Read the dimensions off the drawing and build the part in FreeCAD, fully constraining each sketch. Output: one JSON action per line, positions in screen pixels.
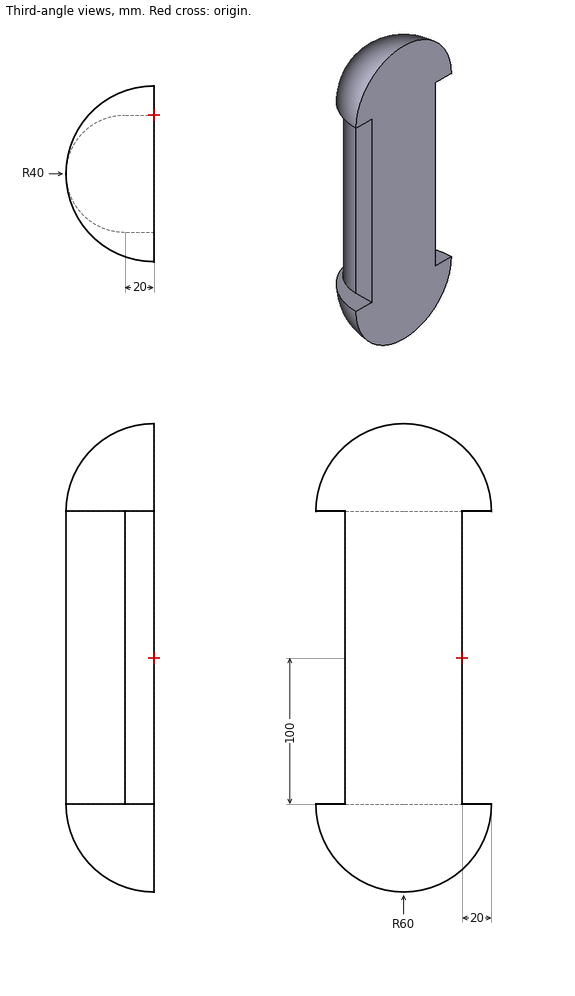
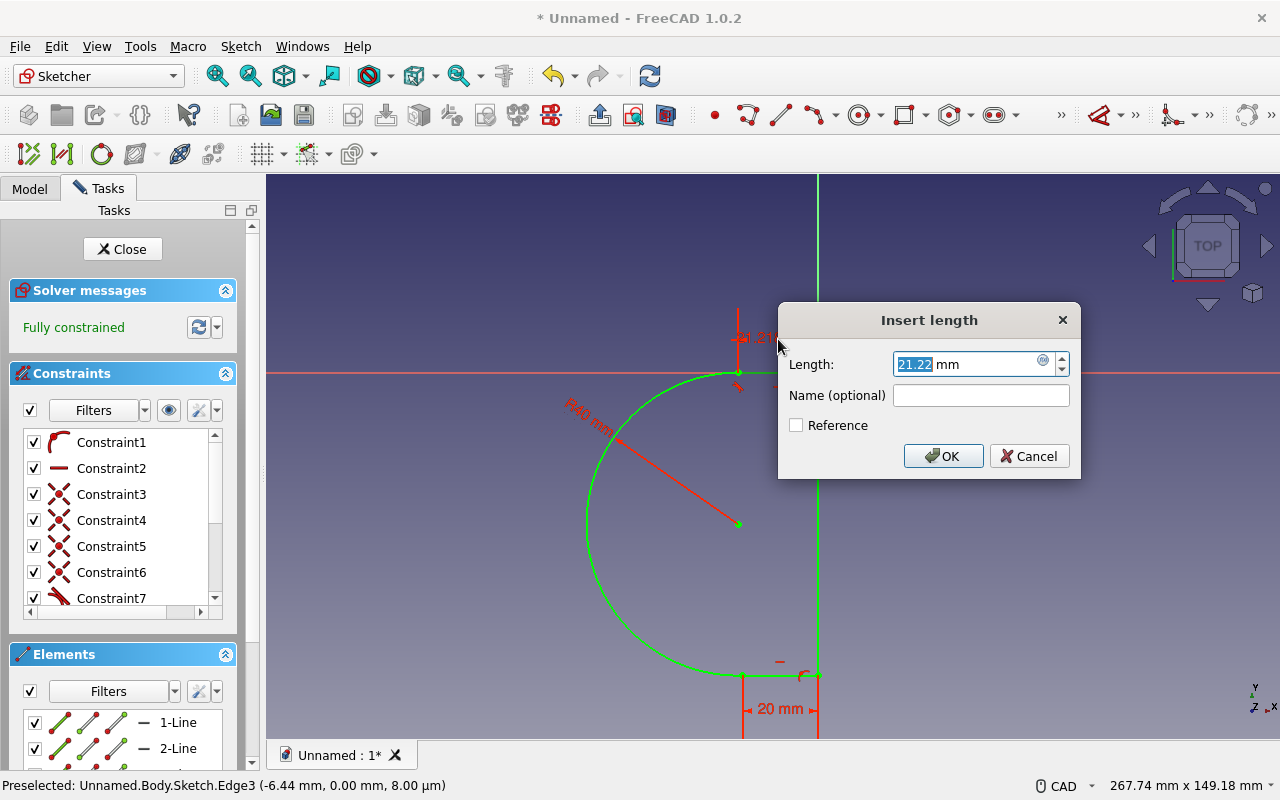
{"action": "type", "text": "20"}
{"action": "key", "text": "Return"}
{"action": "key", "text": "Escape"}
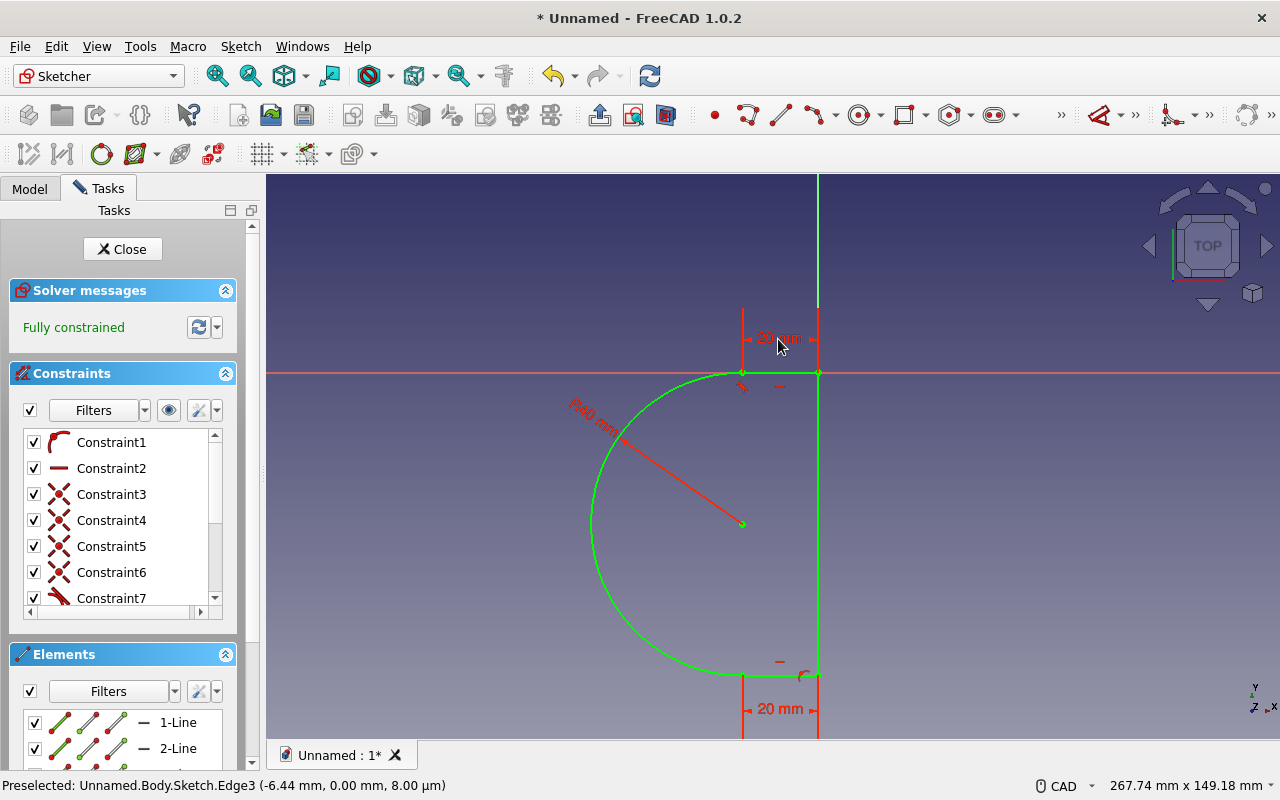
{"action": "left_click", "coordinate": [123, 249]}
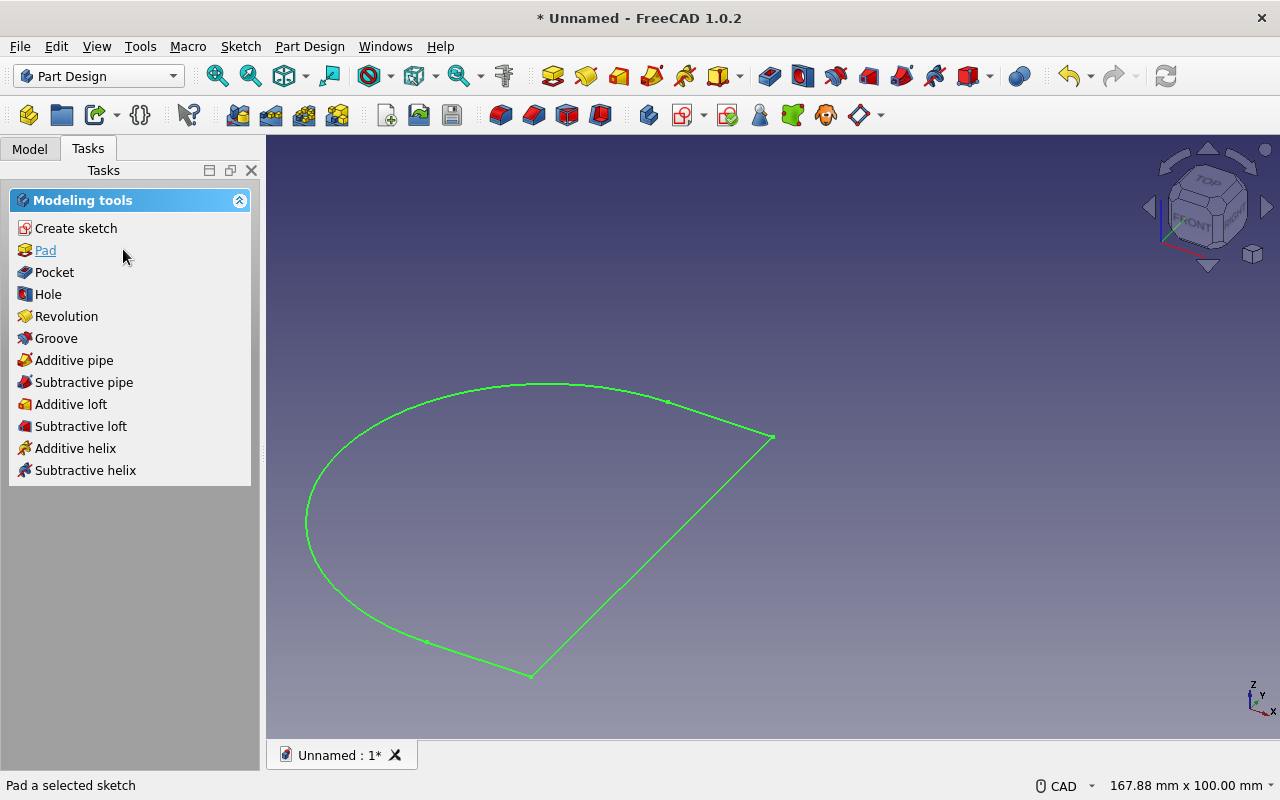
{"action": "left_click", "coordinate": [553, 76]}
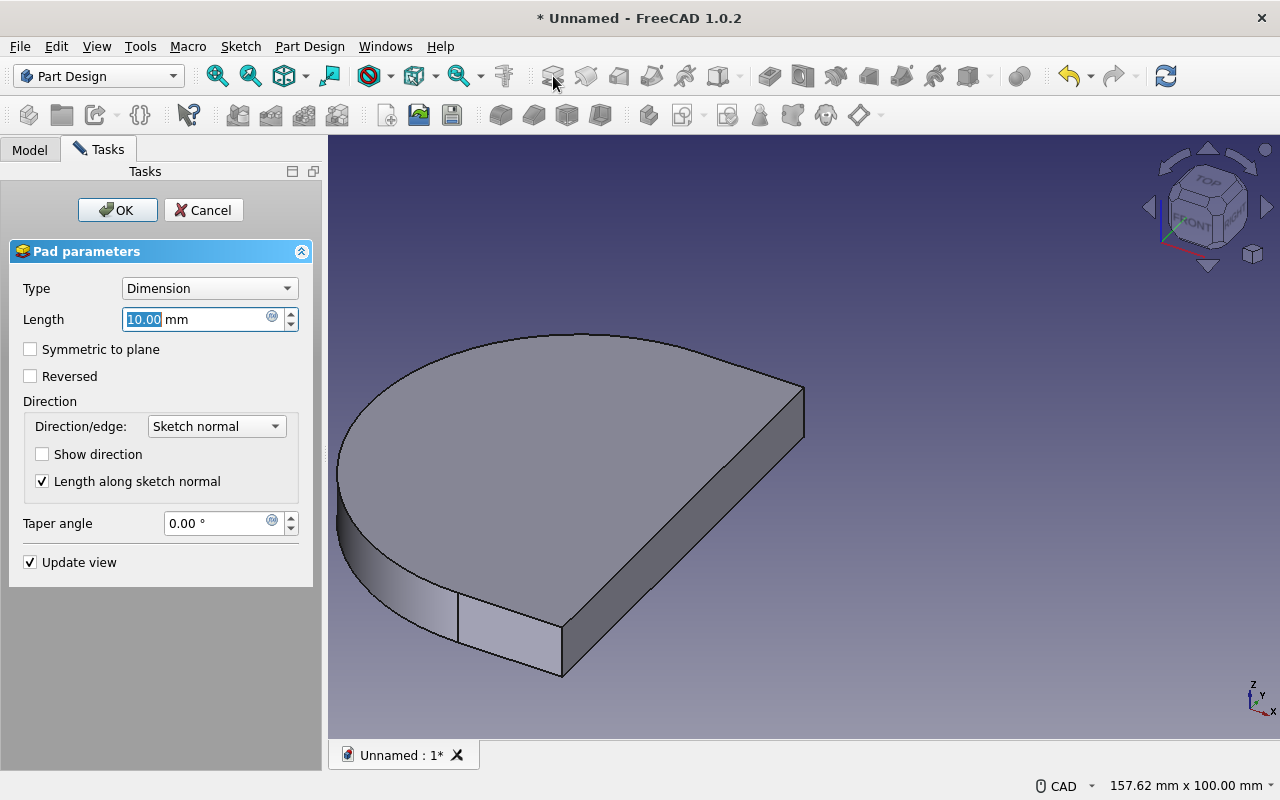
{"action": "type", "text": "100"}
{"action": "key", "text": "Tab"}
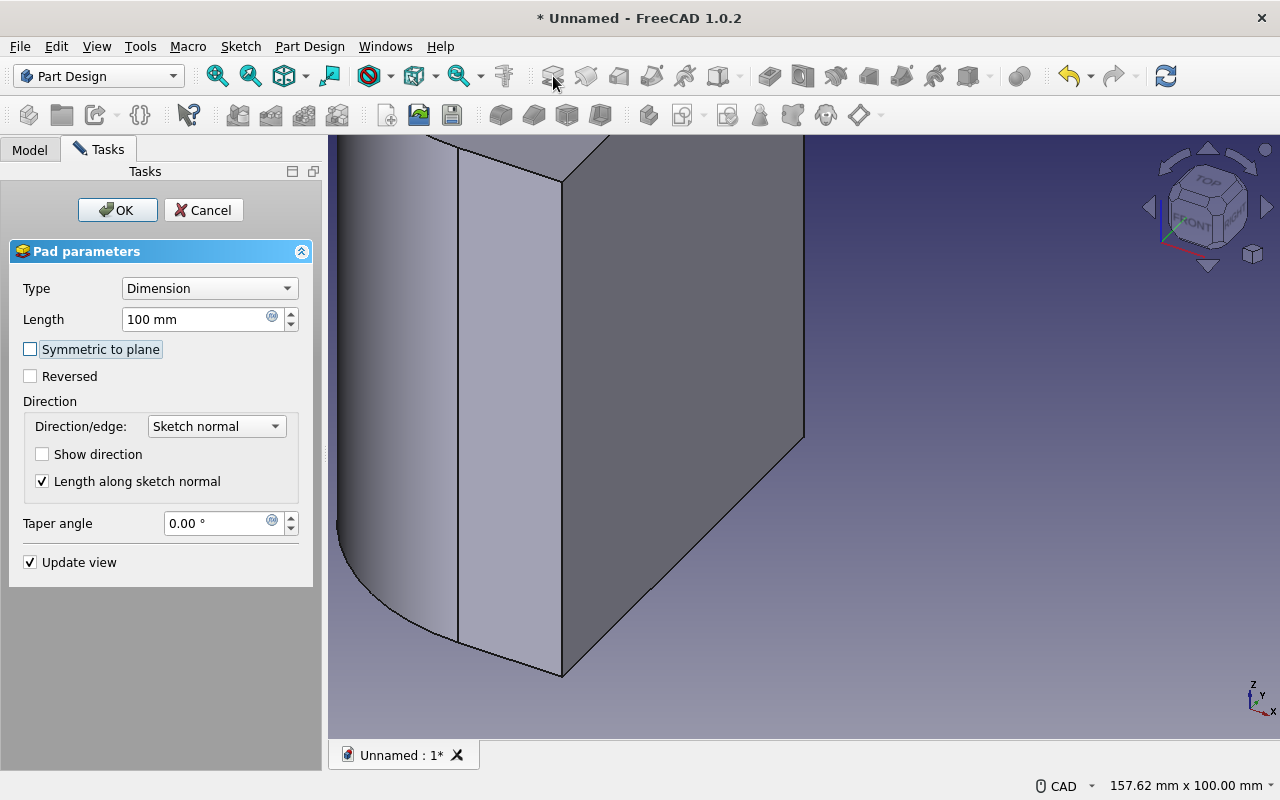
{"action": "left_click", "coordinate": [31, 376]}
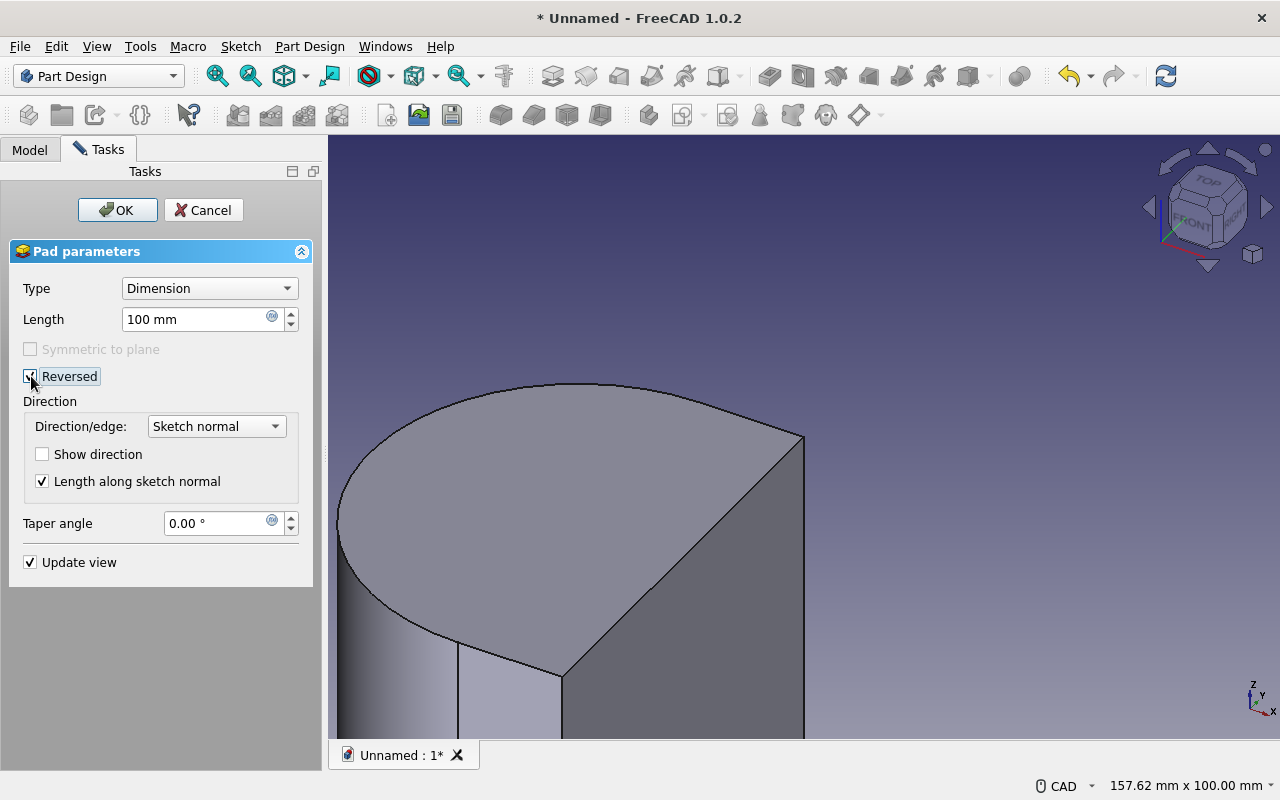
{"action": "left_click", "coordinate": [118, 210]}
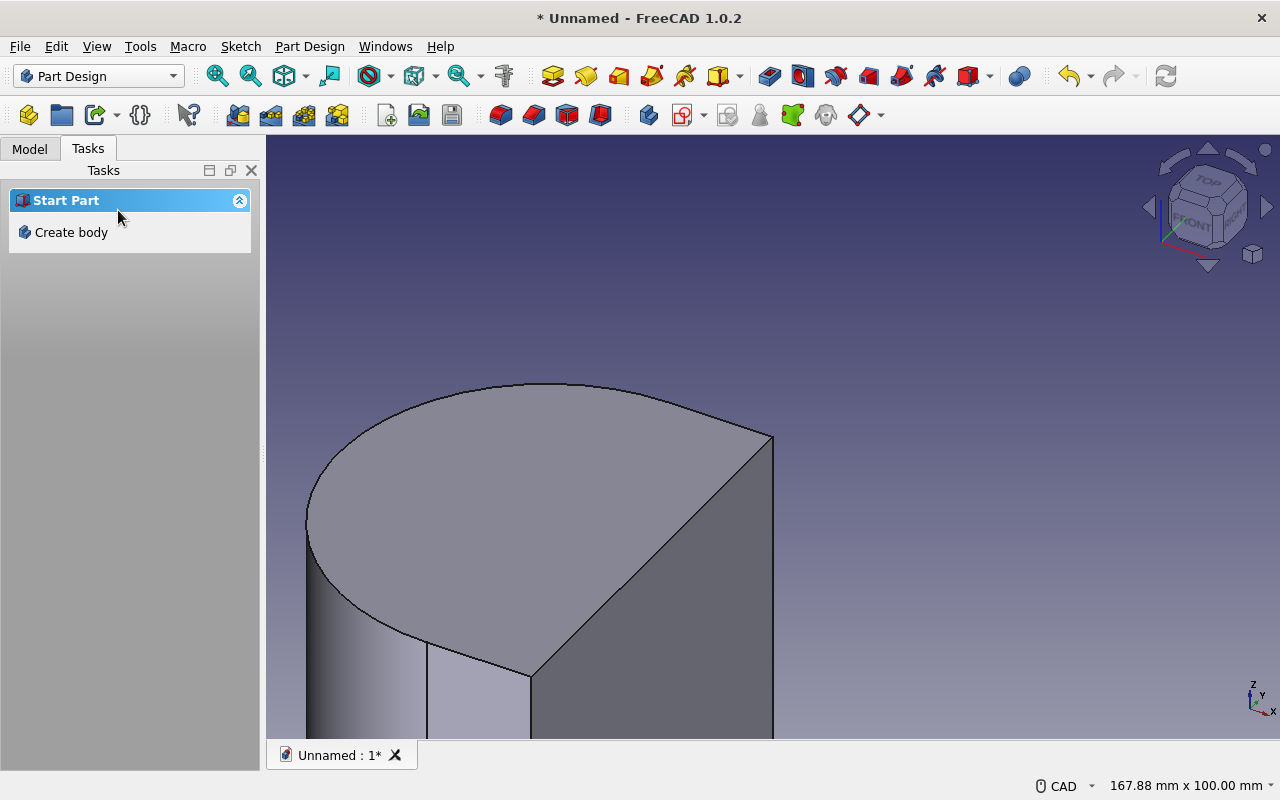
{"action": "key", "text": "v f"}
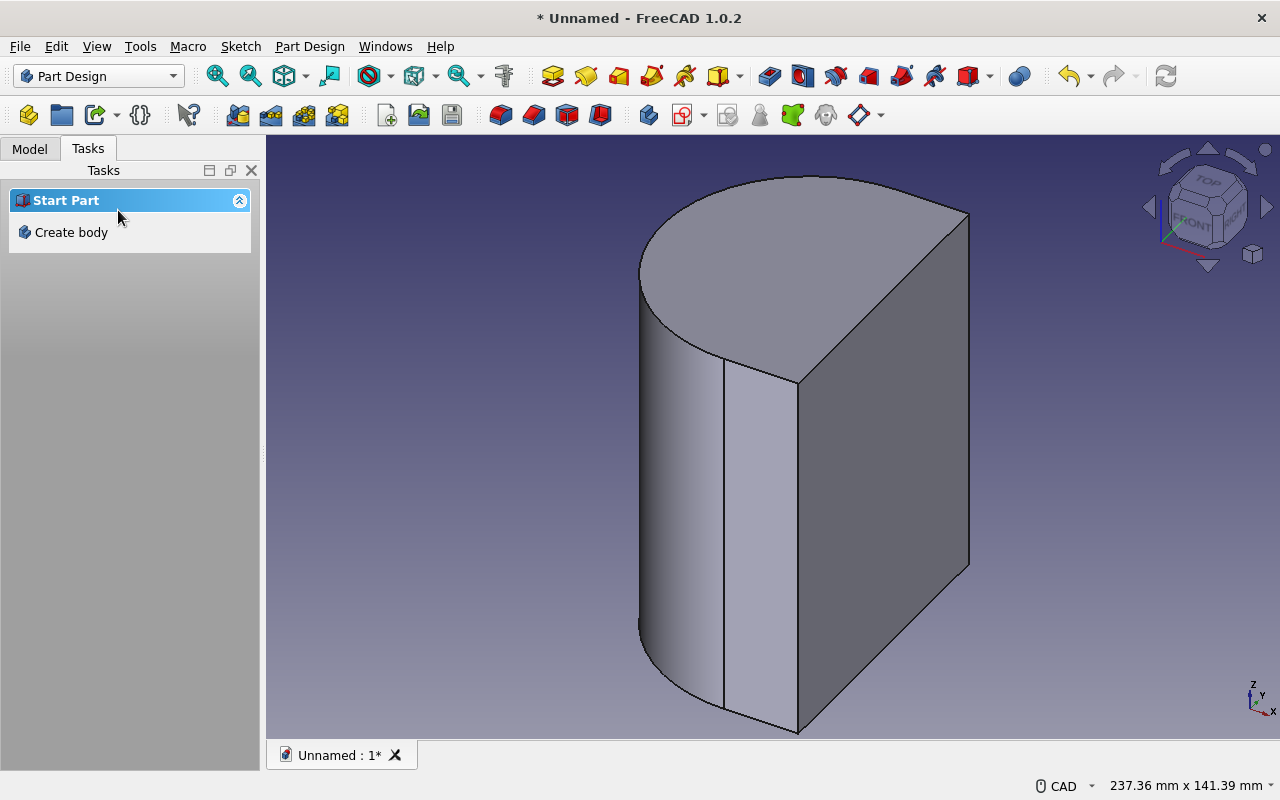
{"action": "left_click", "coordinate": [682, 116]}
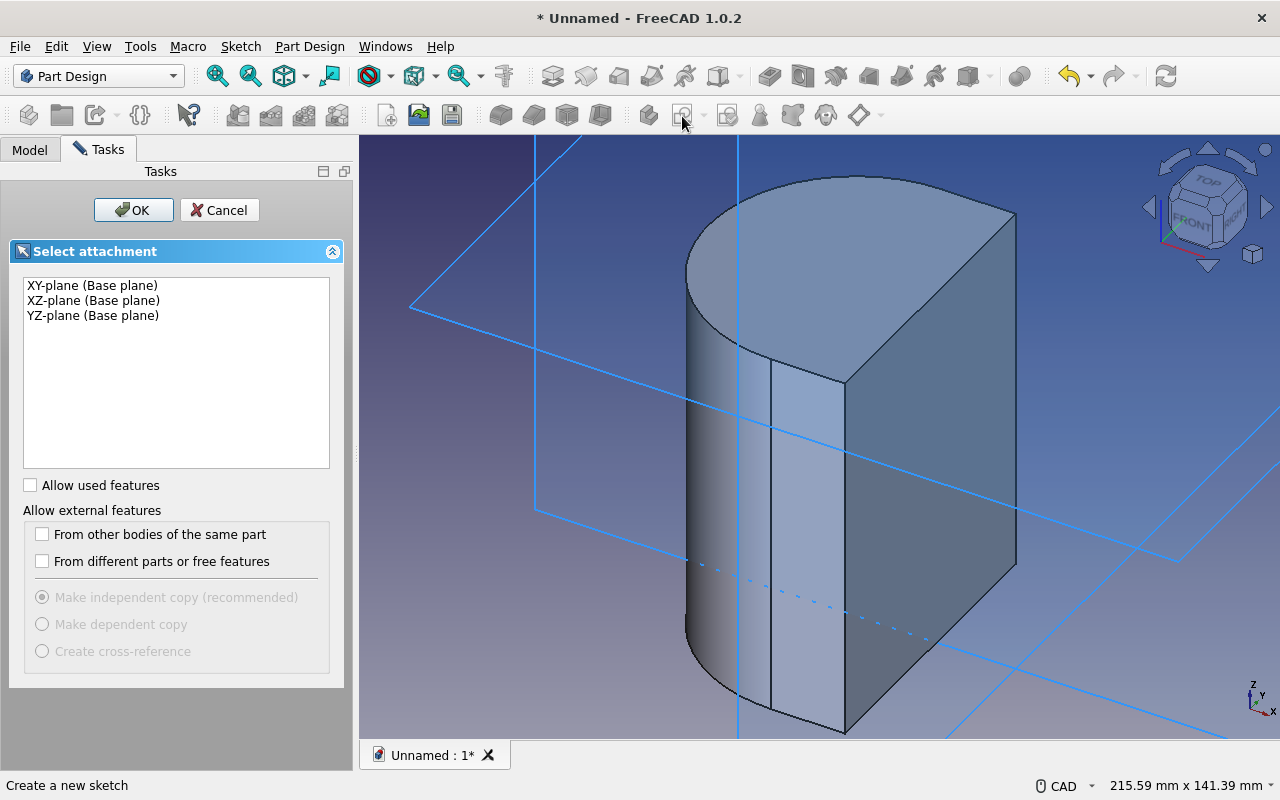
{"action": "left_click", "coordinate": [84, 316]}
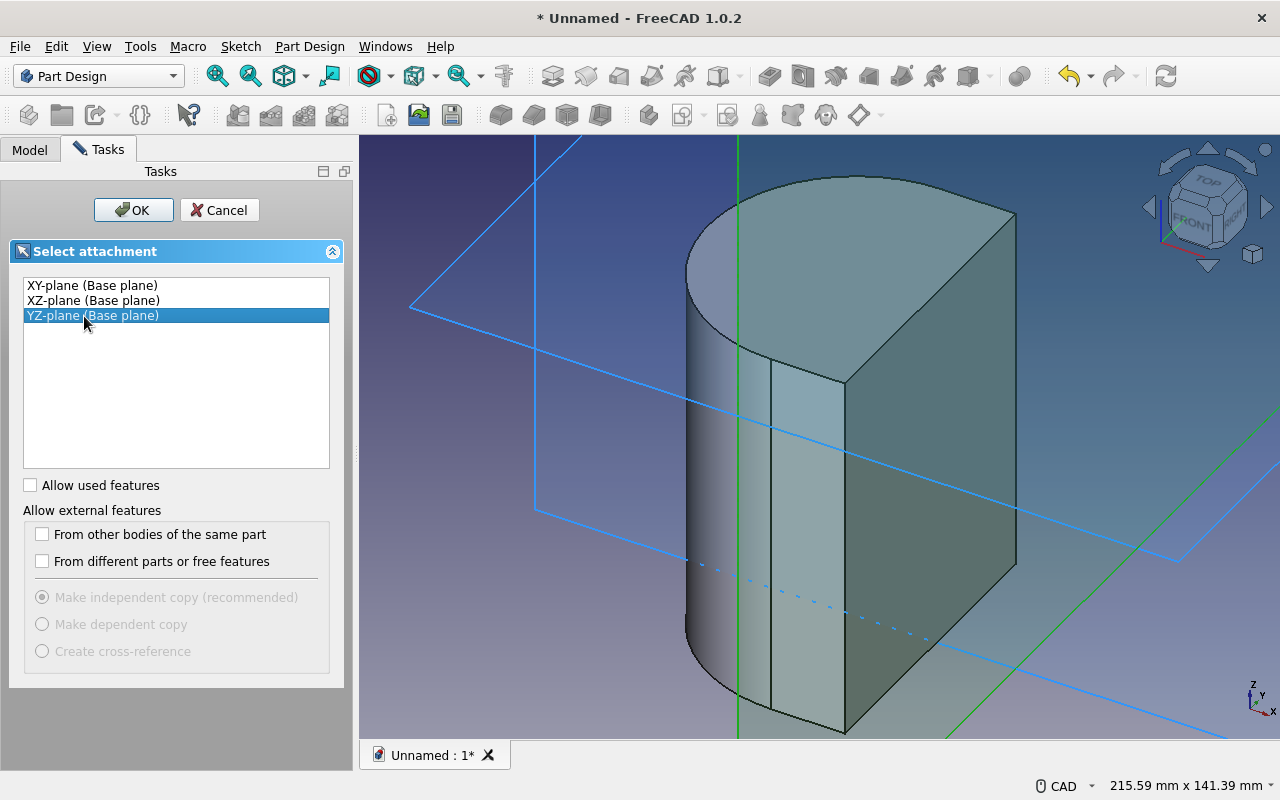
{"action": "left_click", "coordinate": [134, 210]}